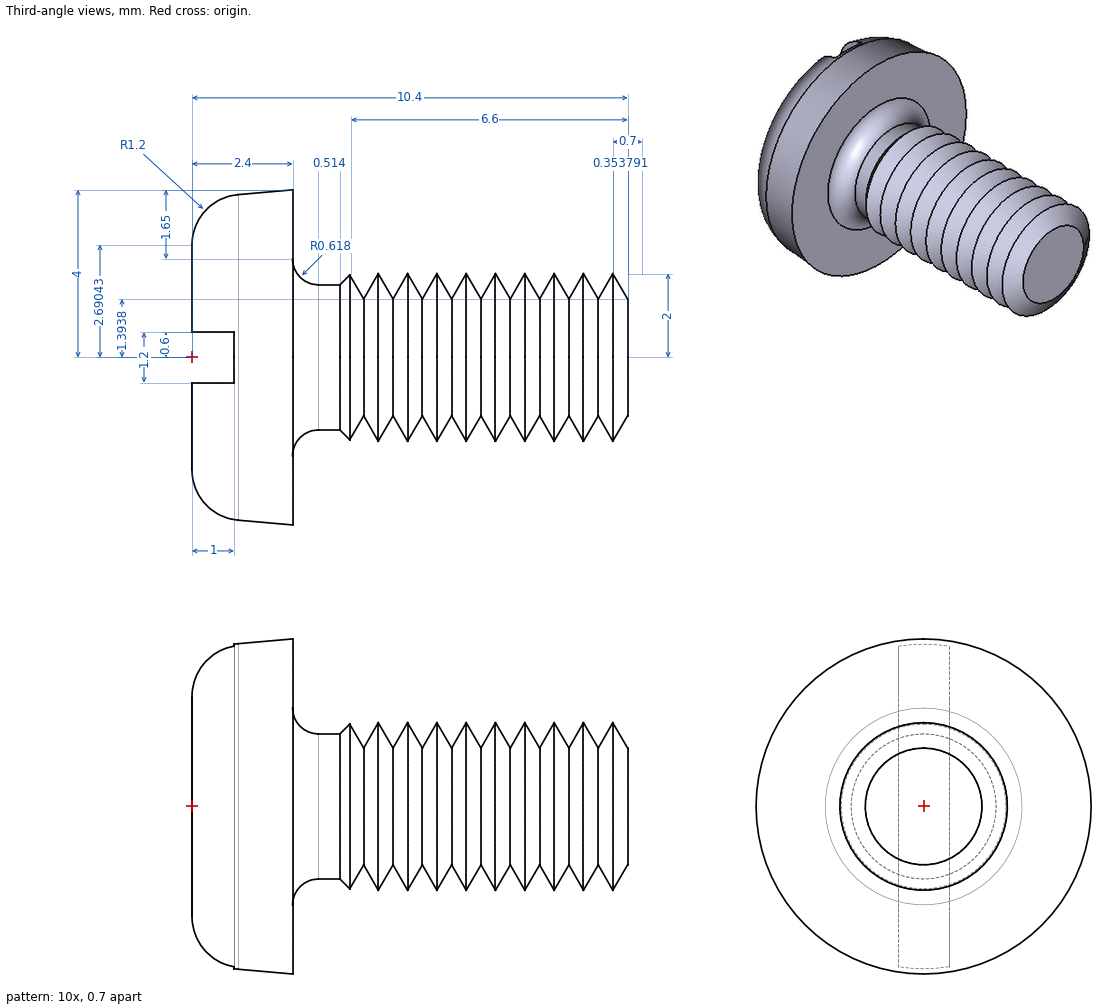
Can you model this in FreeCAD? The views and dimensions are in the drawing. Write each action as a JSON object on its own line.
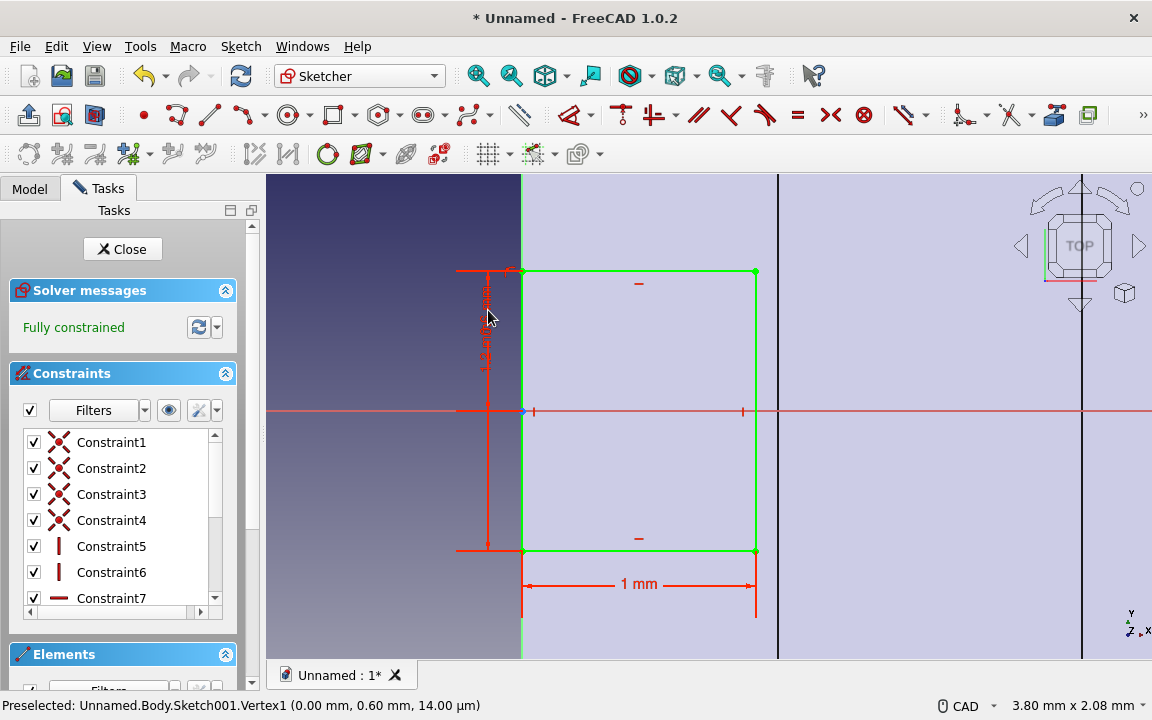
{"action": "left_click", "coordinate": [123, 249]}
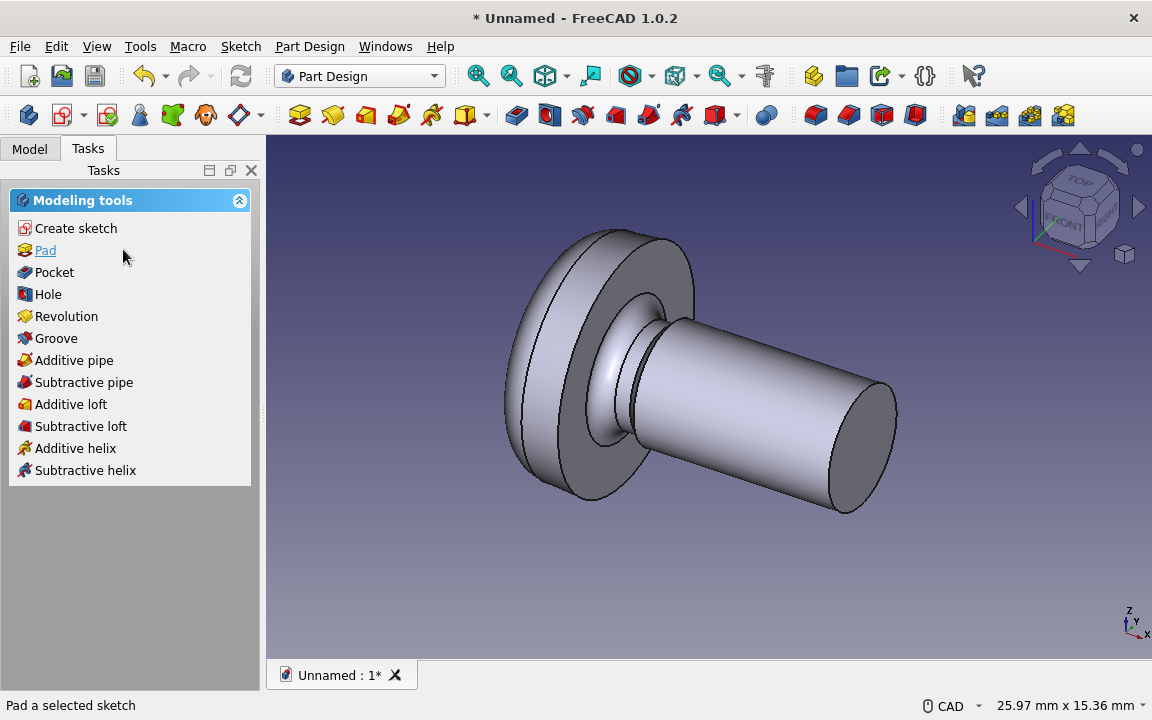
{"action": "left_click", "coordinate": [517, 116]}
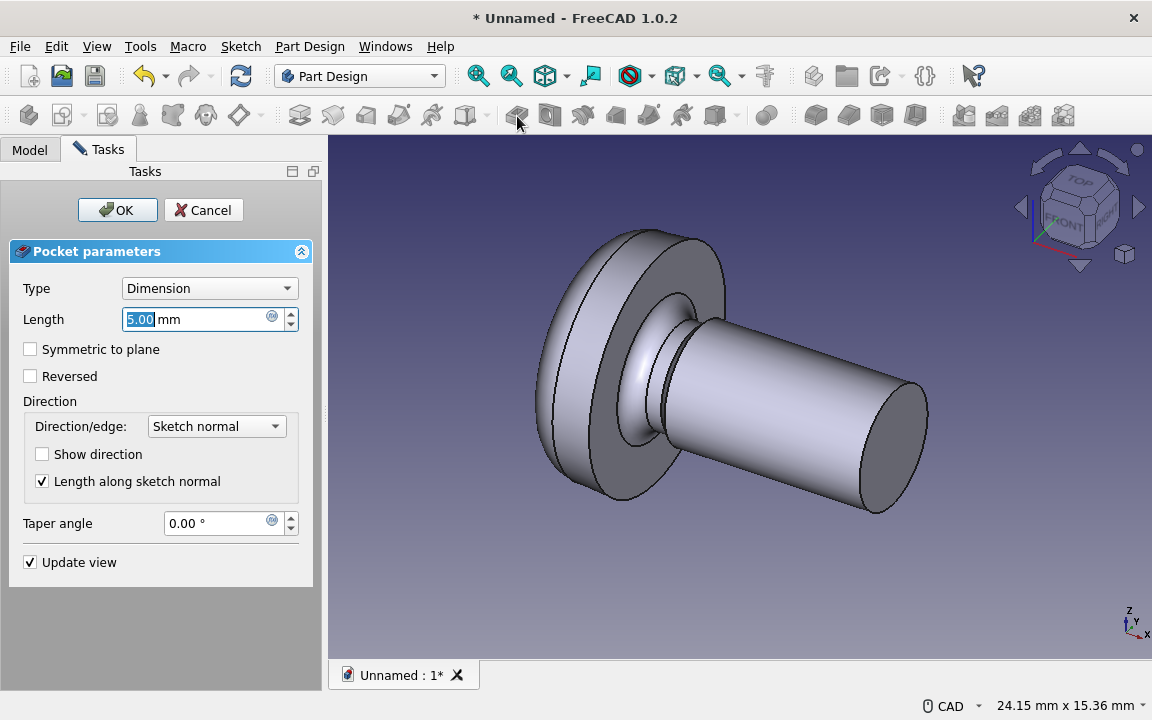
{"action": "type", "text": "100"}
{"action": "key", "text": "Tab"}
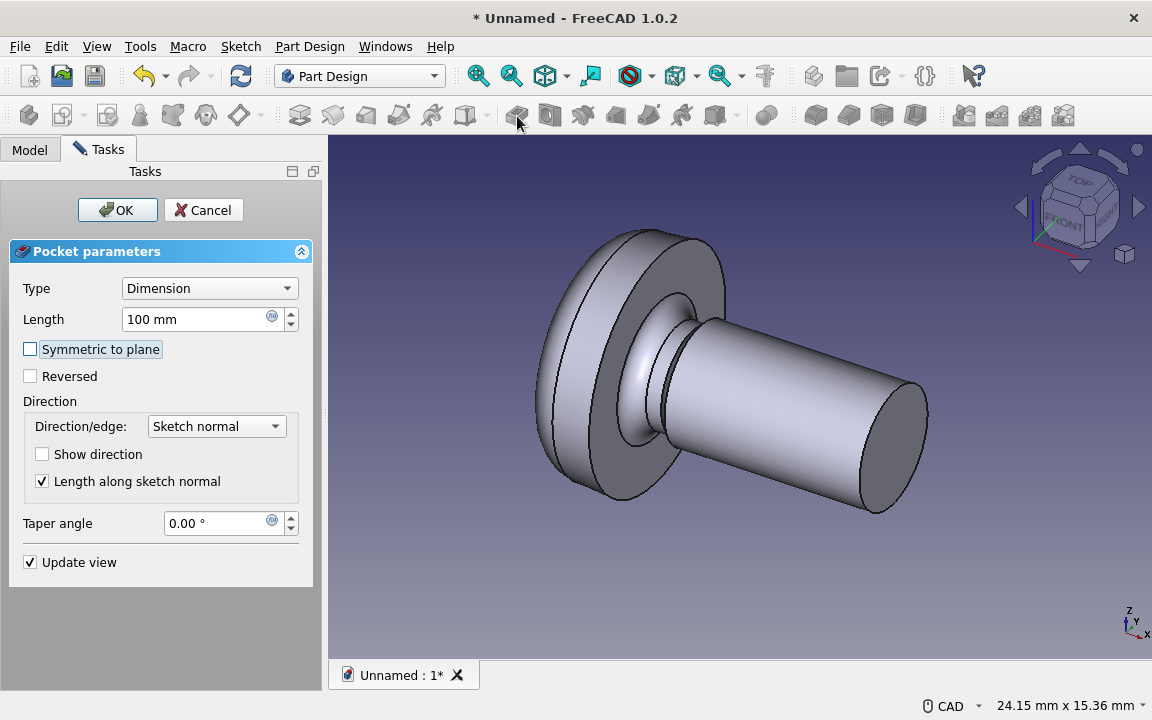
{"action": "left_click", "coordinate": [31, 349]}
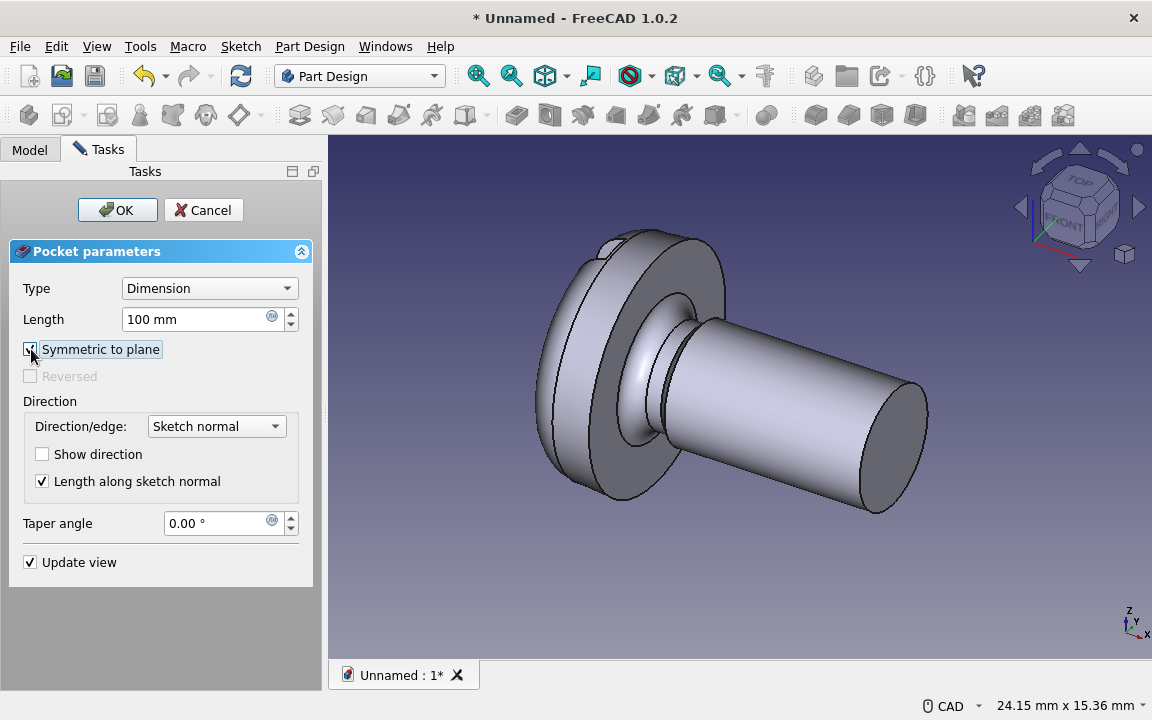
{"action": "left_click", "coordinate": [118, 210]}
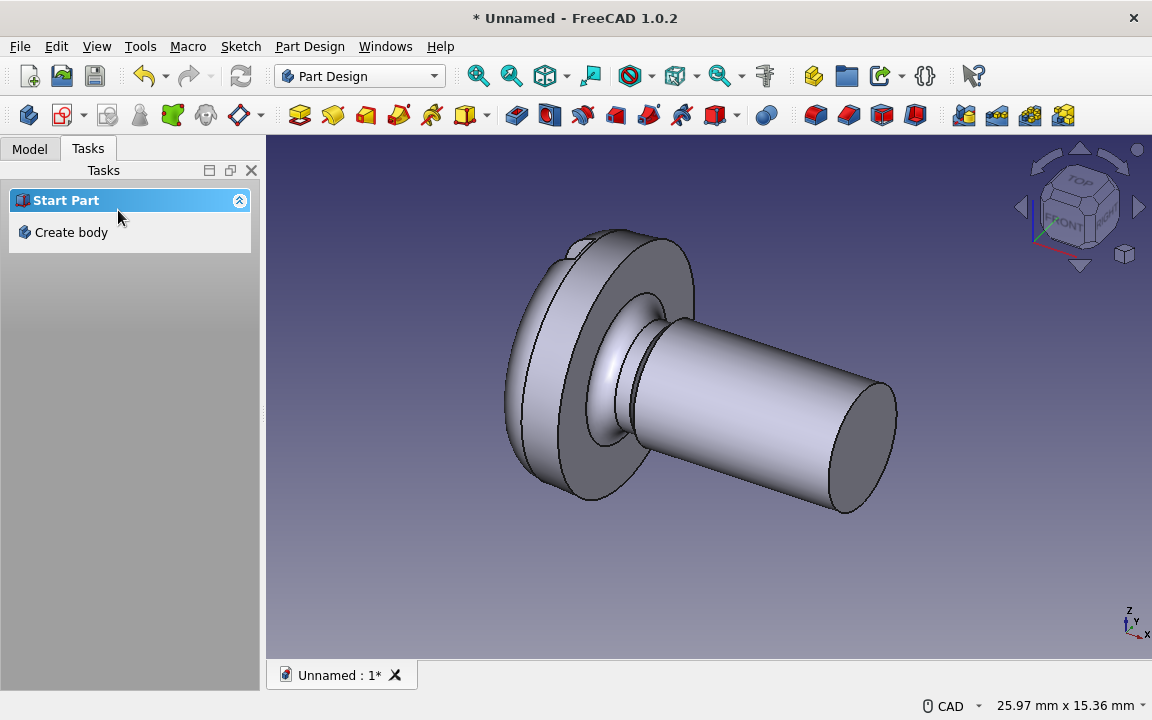
{"action": "left_click", "coordinate": [62, 116]}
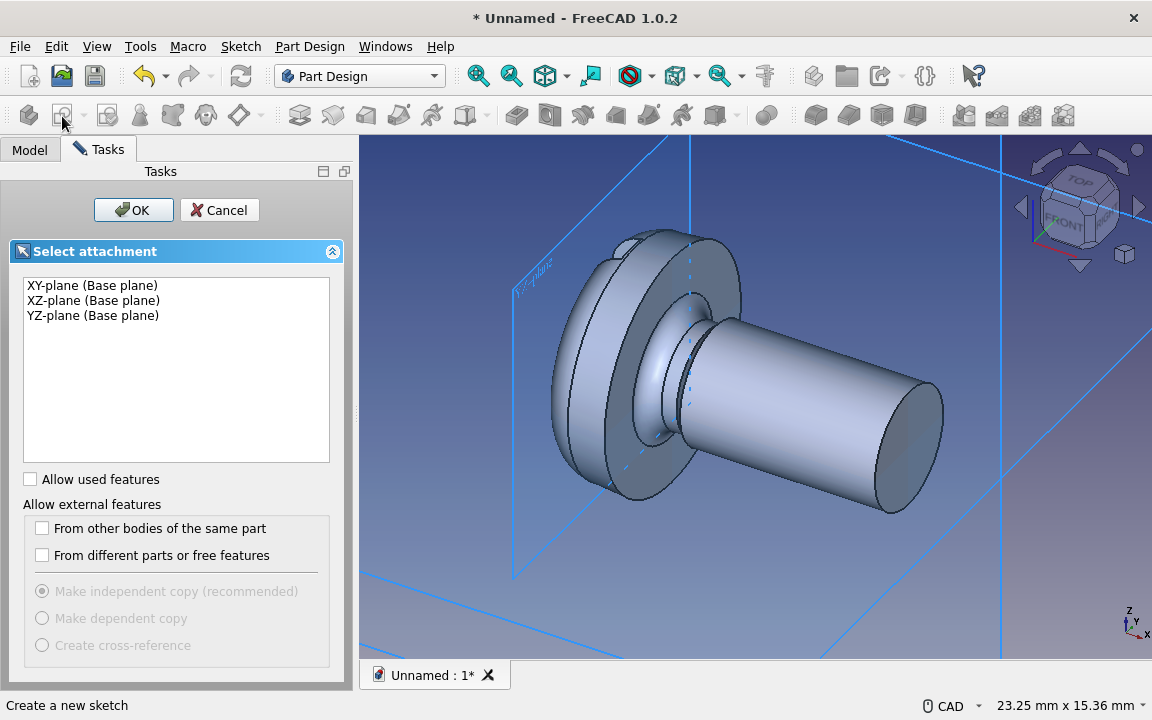
{"action": "left_click", "coordinate": [84, 286]}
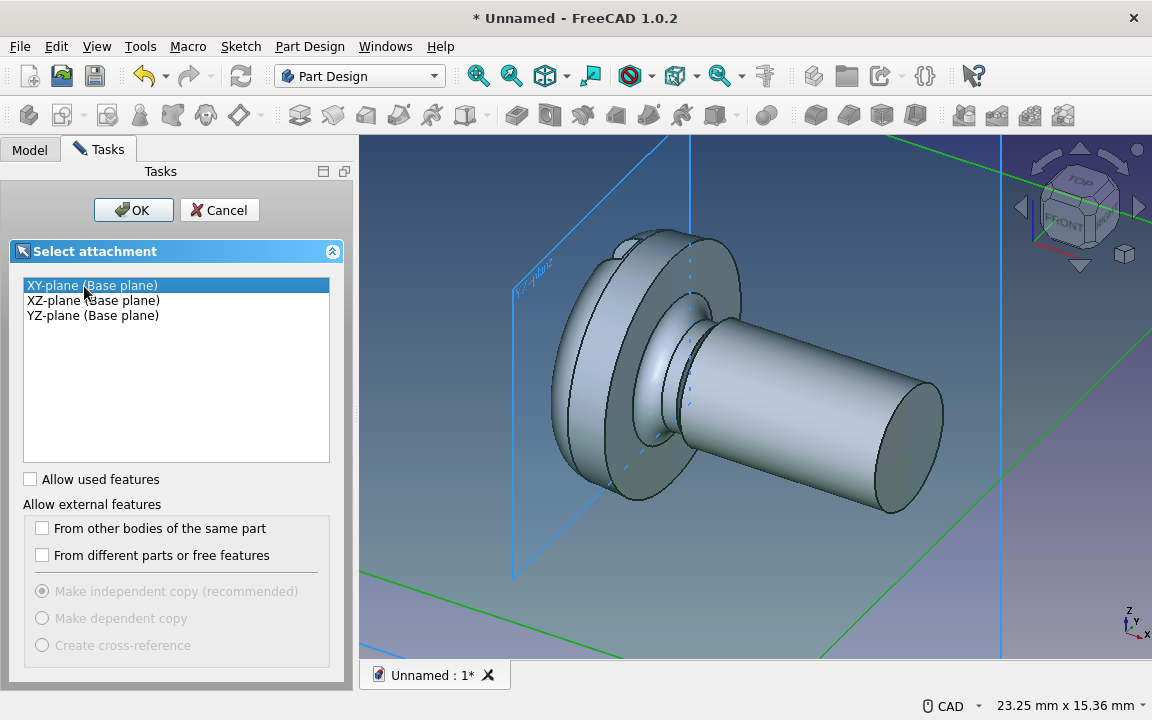
{"action": "left_click", "coordinate": [134, 210]}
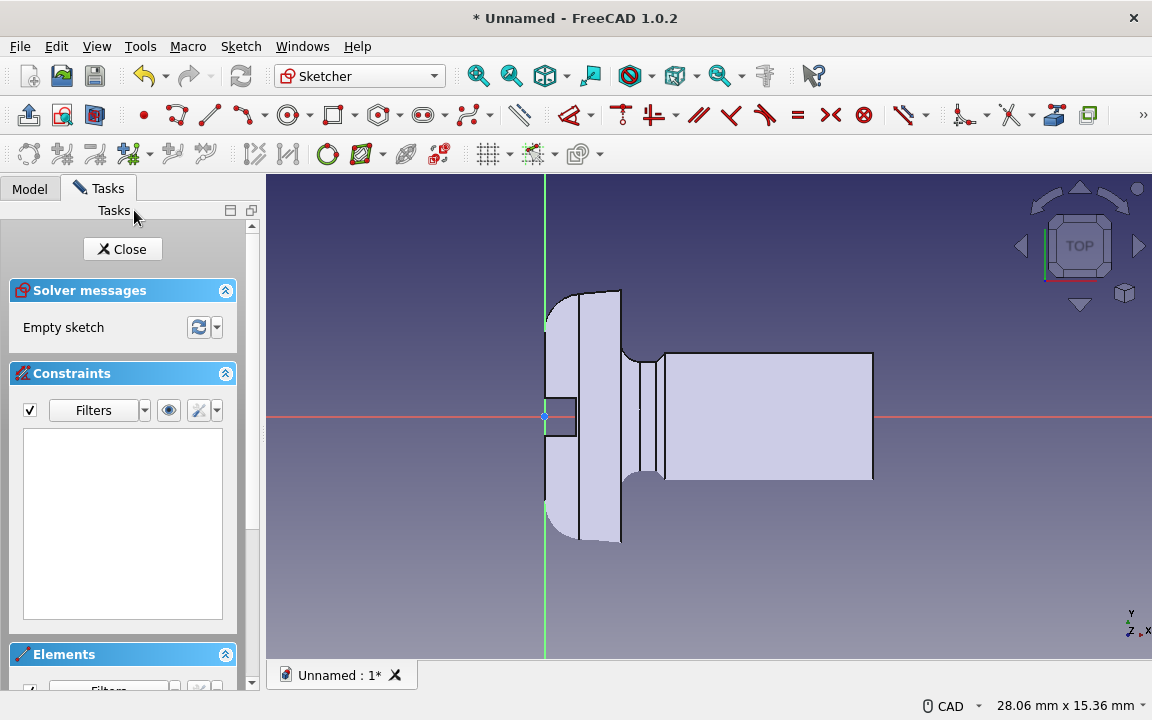
{"action": "left_click", "coordinate": [95, 116]}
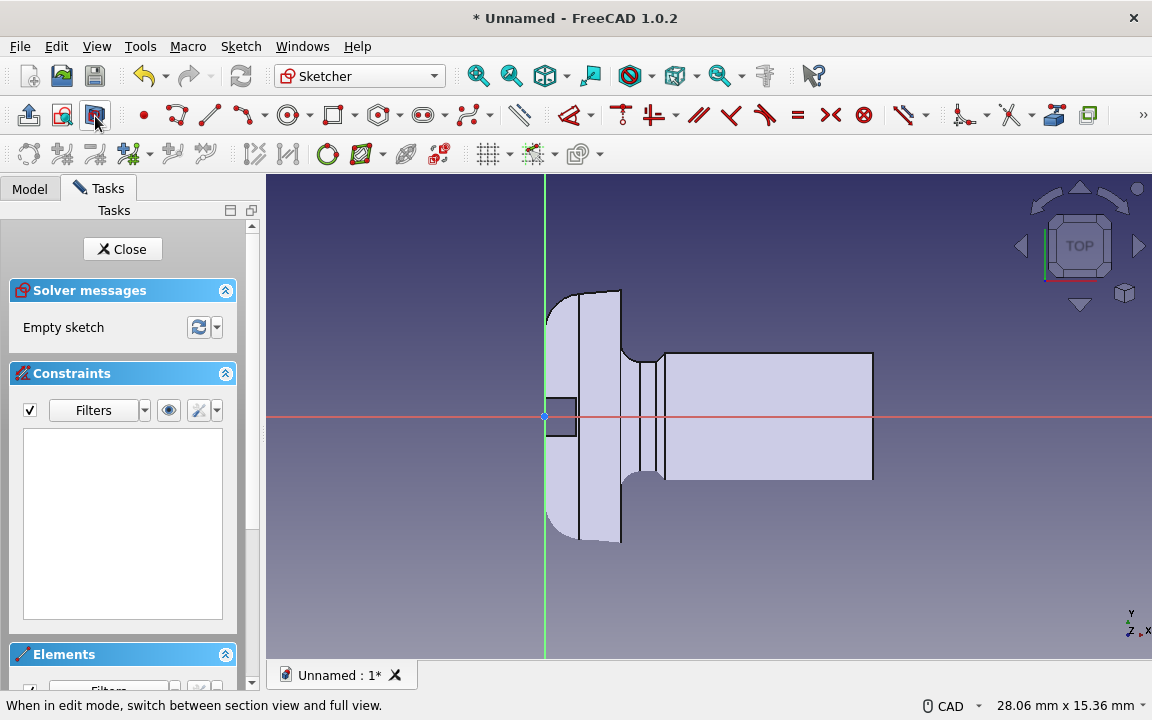
{"action": "scroll", "coordinate": [888, 360], "scroll_direction": "up", "scroll_amount": 14}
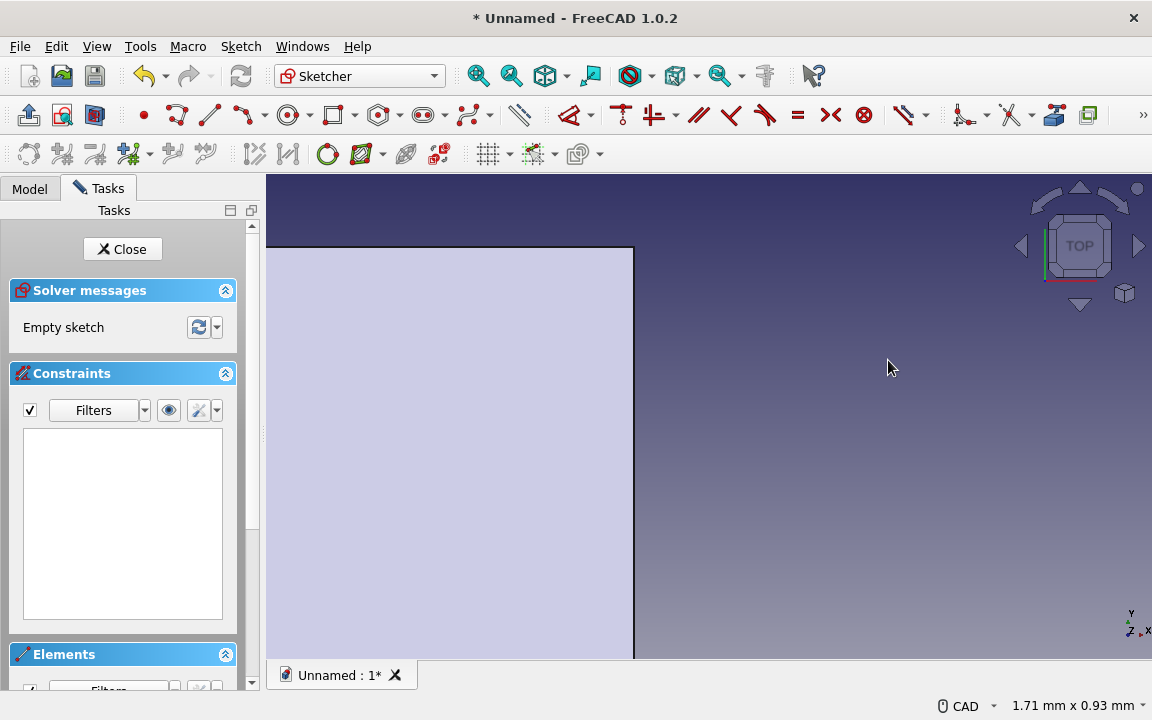
{"action": "left_click", "coordinate": [177, 116]}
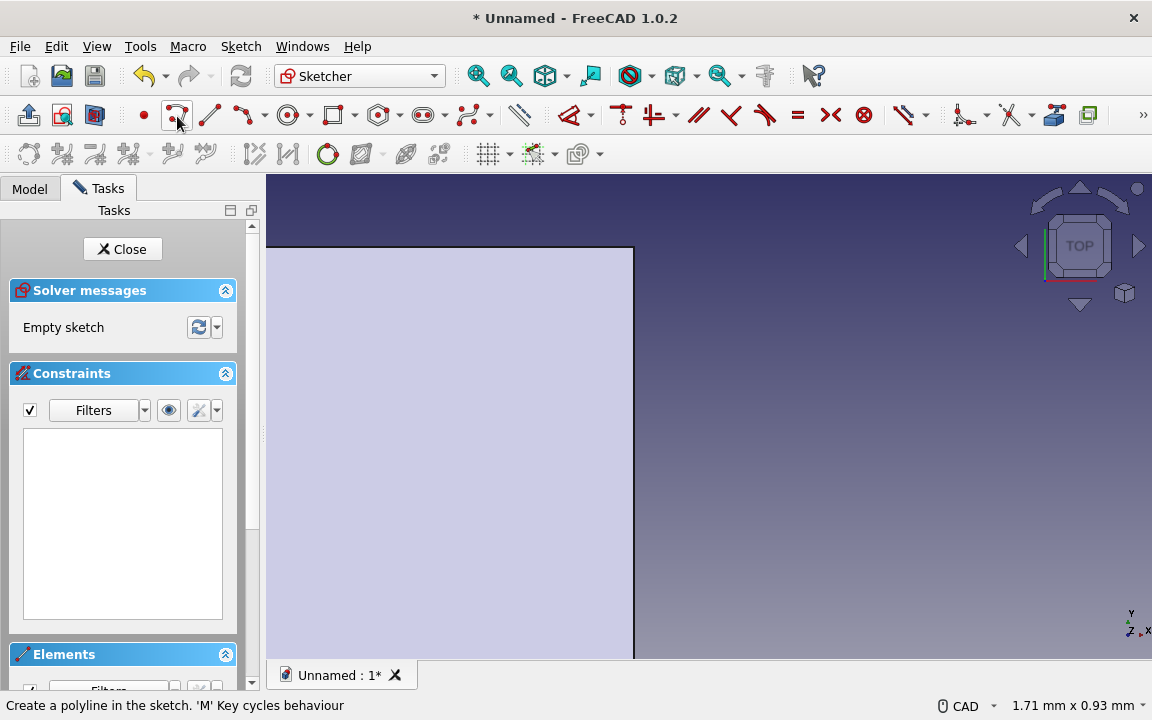
{"action": "left_click", "coordinate": [450, 247]}
{"action": "left_click", "coordinate": [634, 562]}
{"action": "left_click", "coordinate": [813, 247]}
{"action": "left_click", "coordinate": [450, 248]}
{"action": "key", "text": "Escape"}
{"action": "key", "text": "Escape"}